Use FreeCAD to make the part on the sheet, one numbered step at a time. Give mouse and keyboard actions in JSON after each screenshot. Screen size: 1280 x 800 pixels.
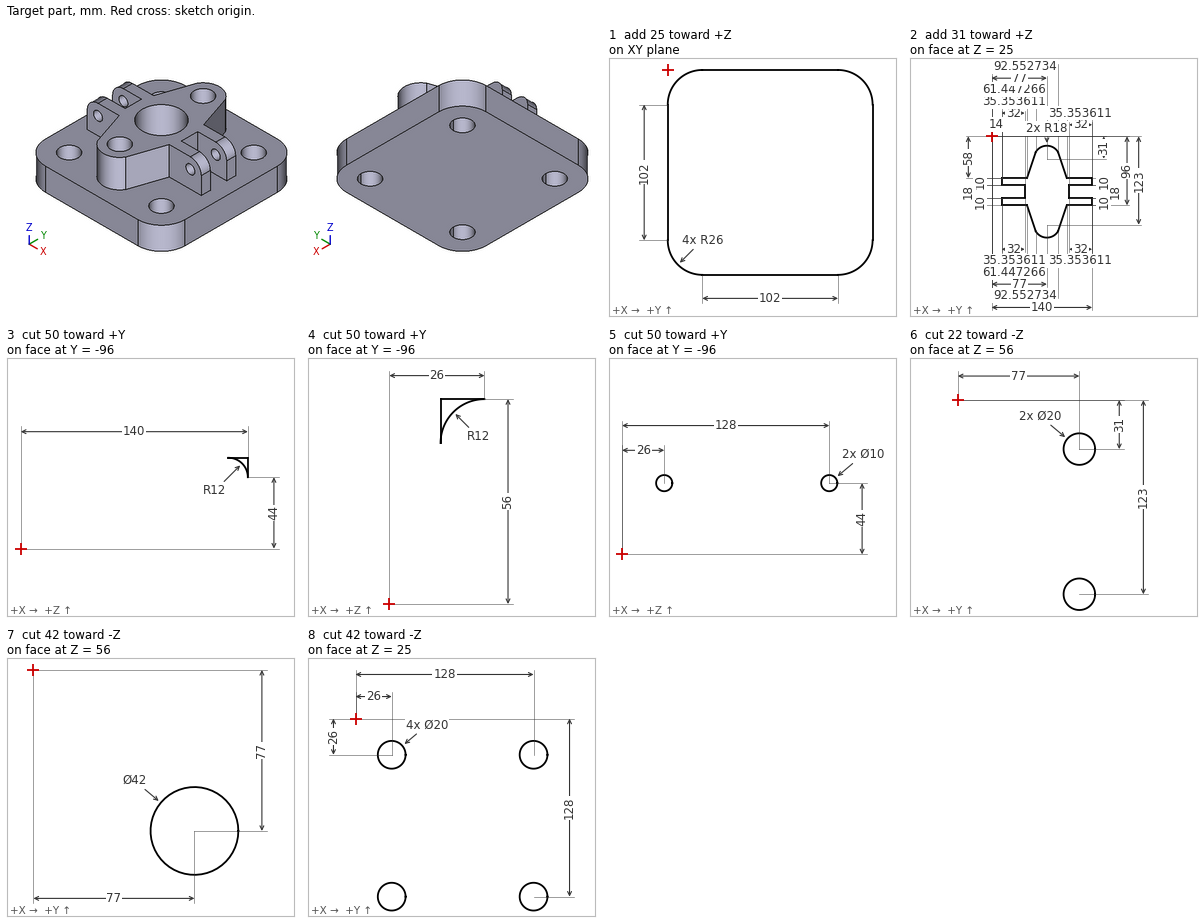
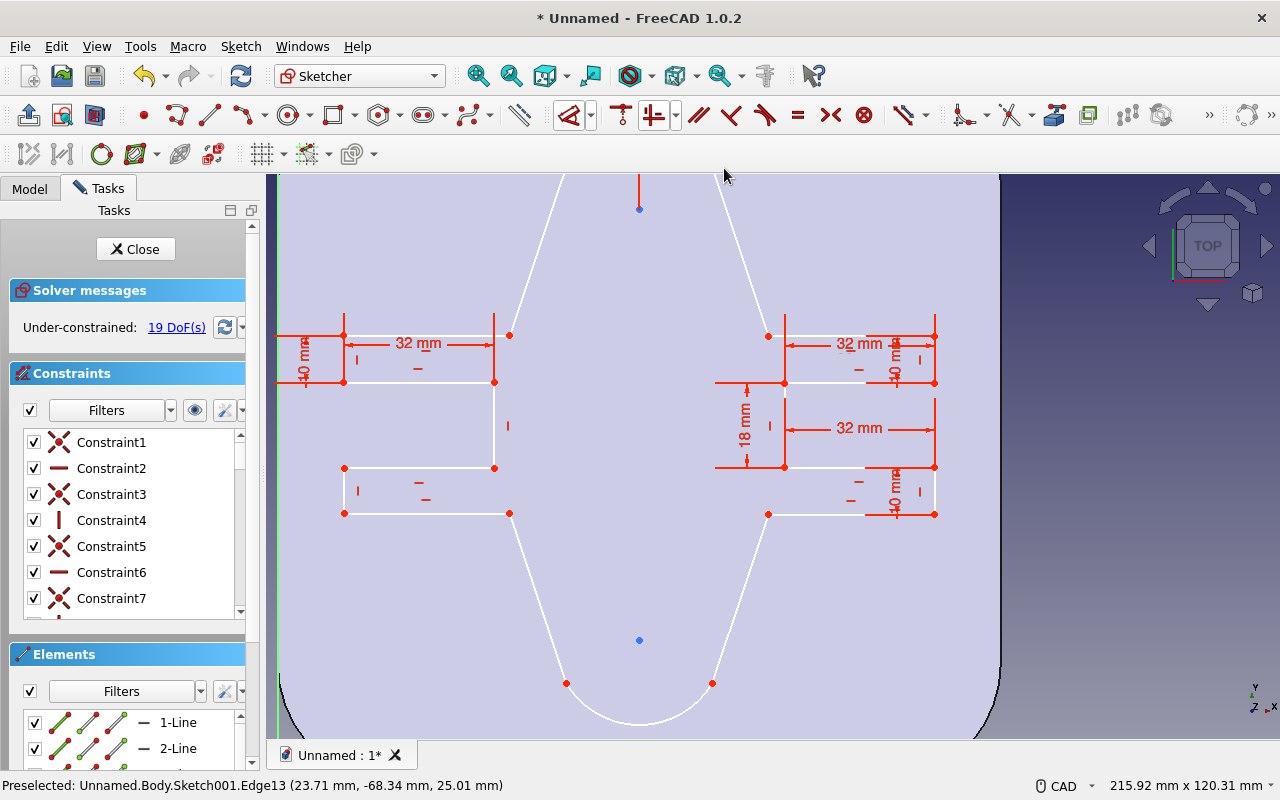
{"action": "left_click", "coordinate": [494, 408]}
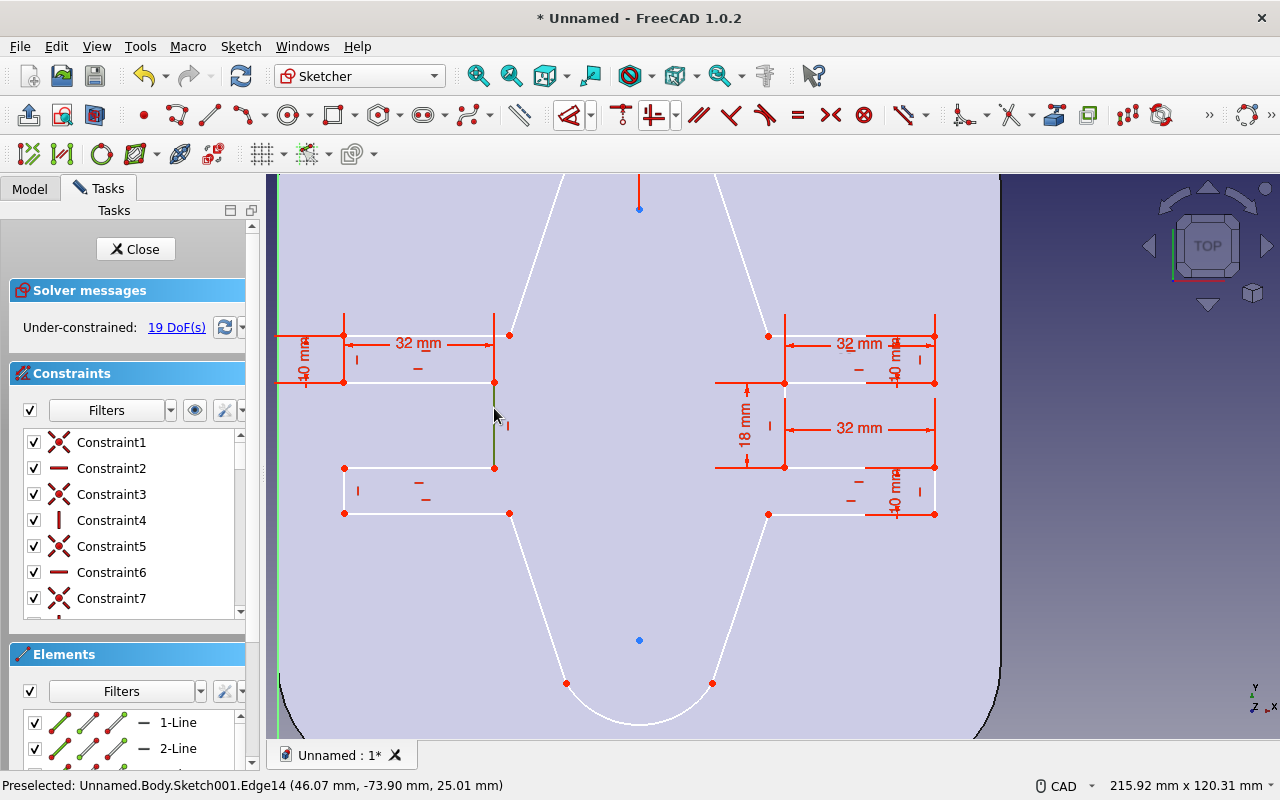
{"action": "left_click", "coordinate": [590, 116]}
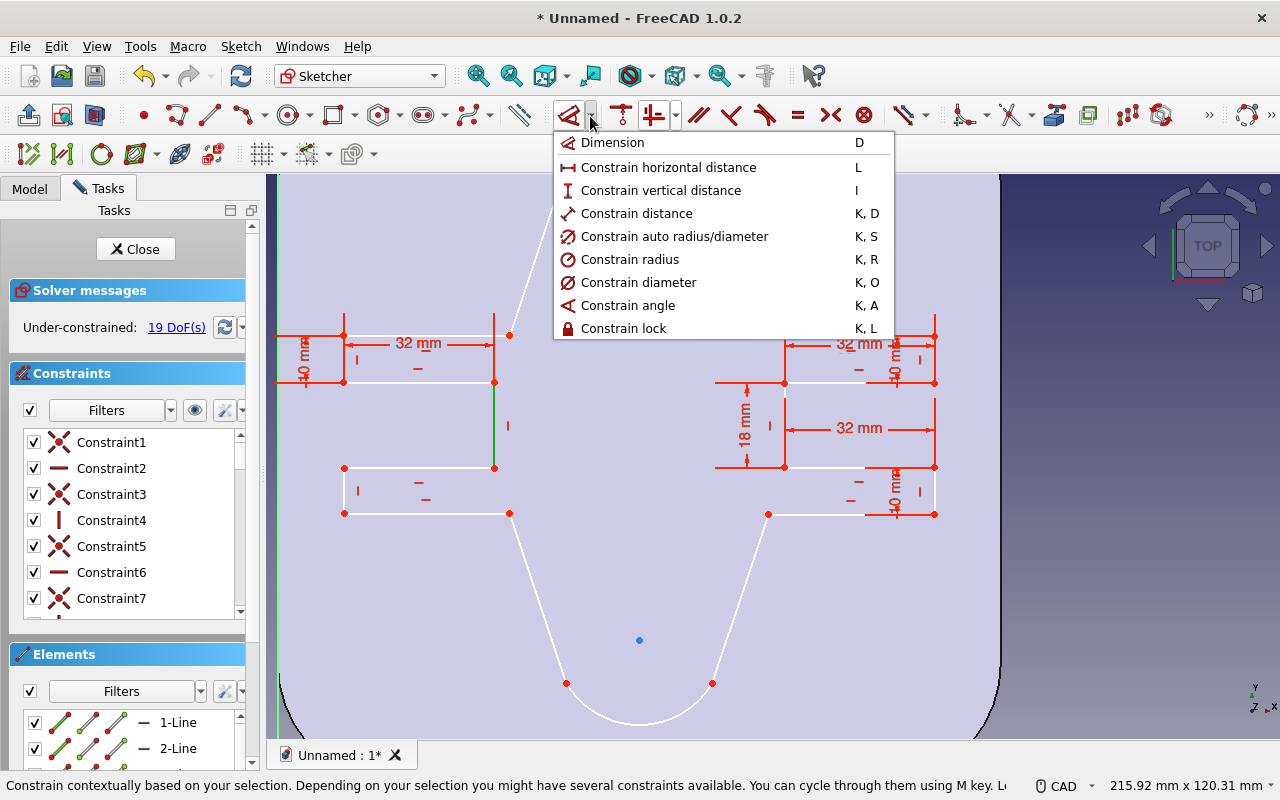
{"action": "left_click", "coordinate": [724, 190]}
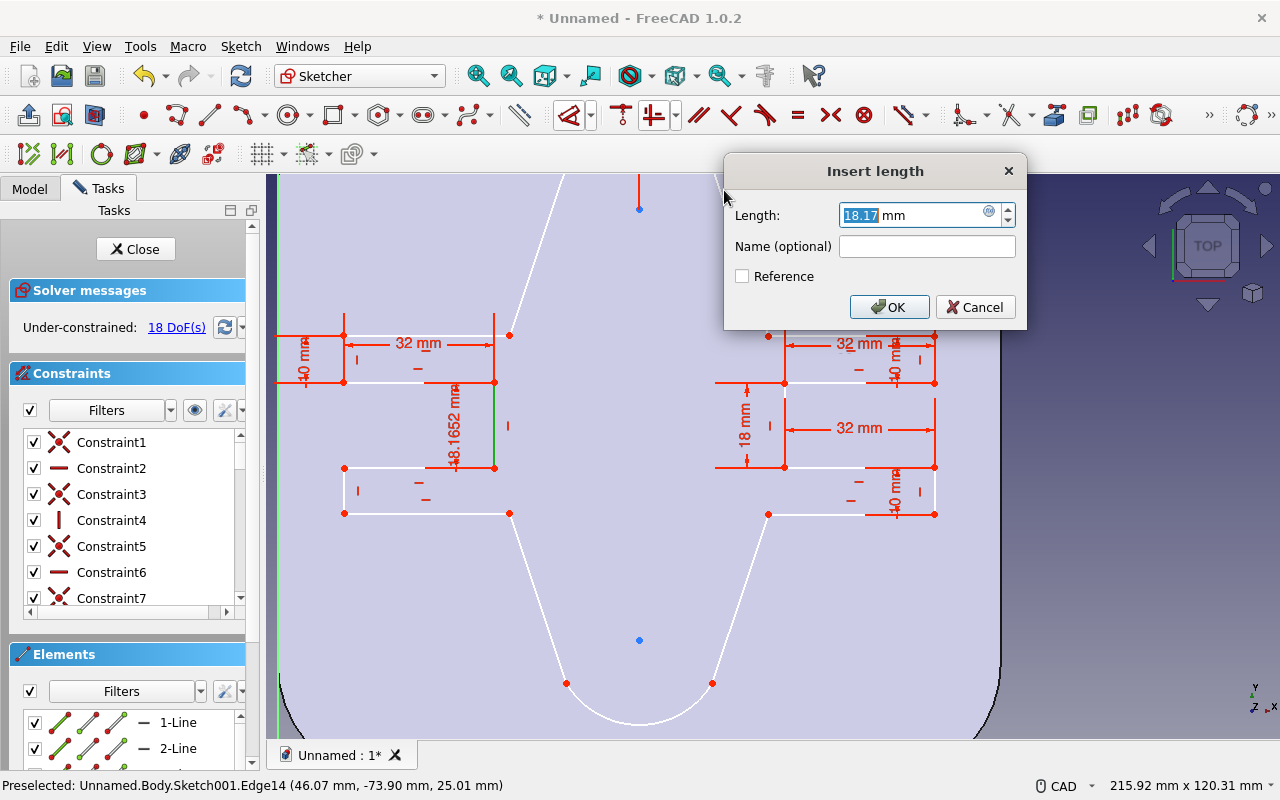
{"action": "type", "text": "18"}
{"action": "key", "text": "Return"}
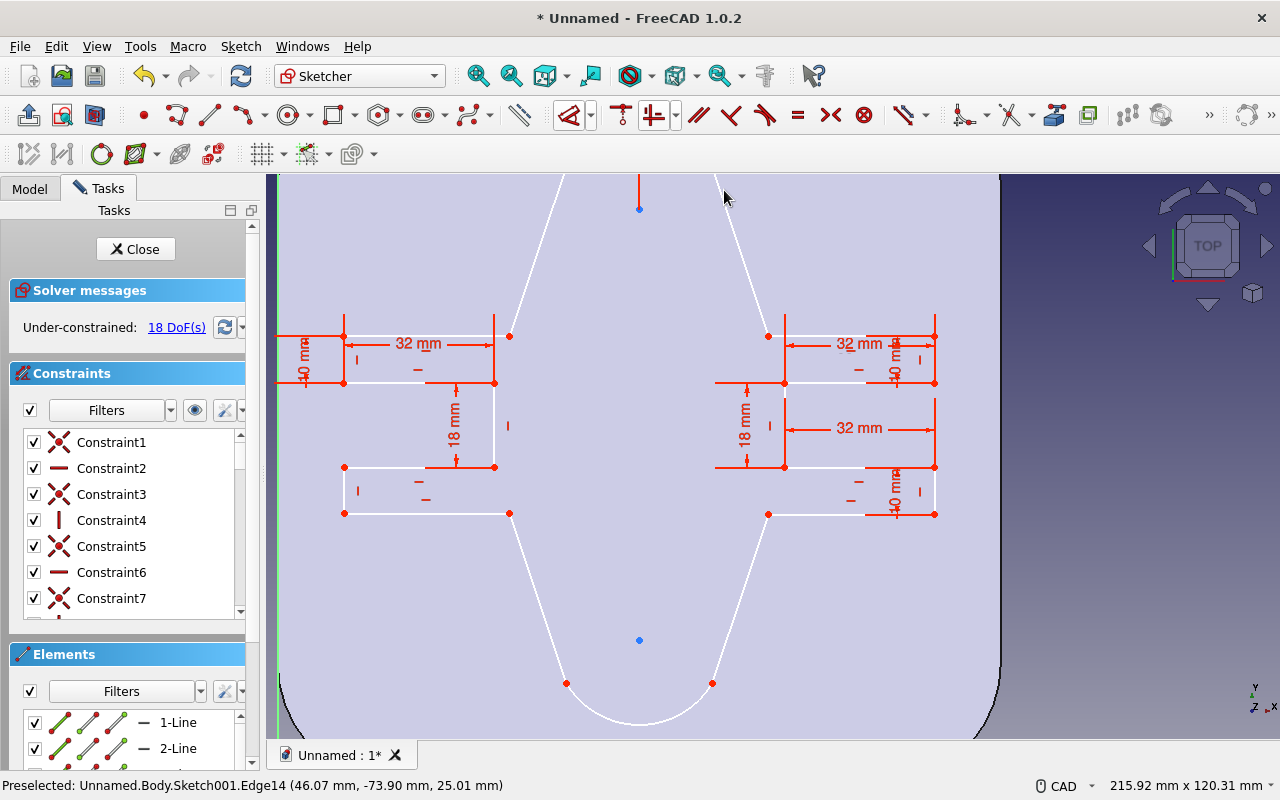
{"action": "left_click", "coordinate": [449, 468]}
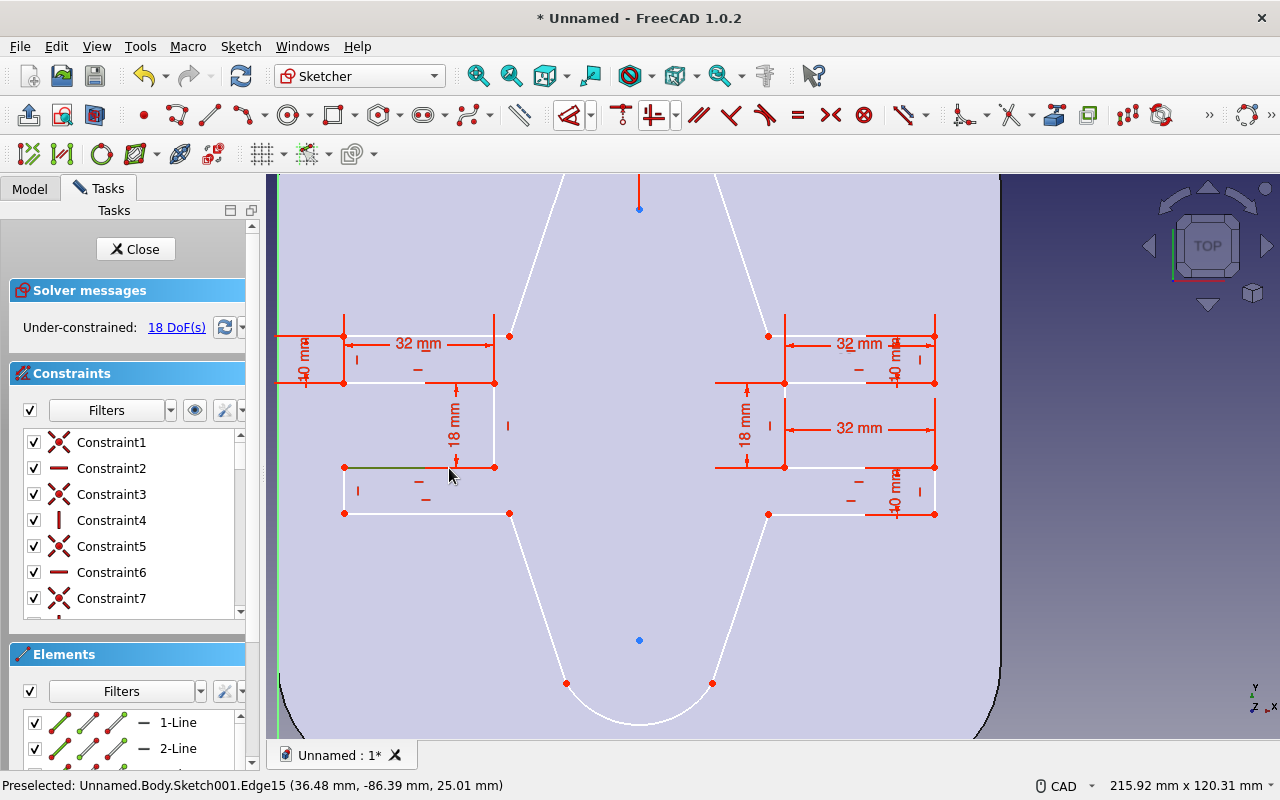
{"action": "key", "text": "l"}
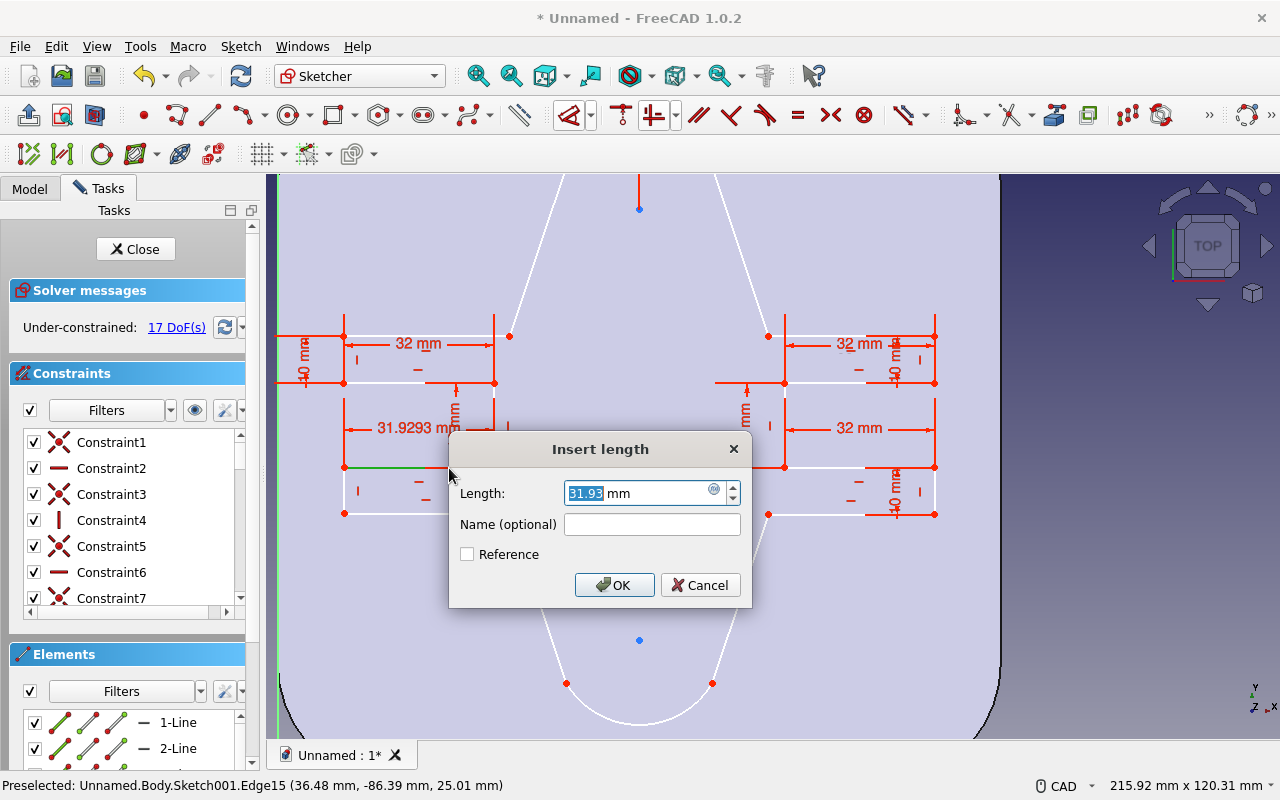
{"action": "type", "text": "32"}
{"action": "key", "text": "Return"}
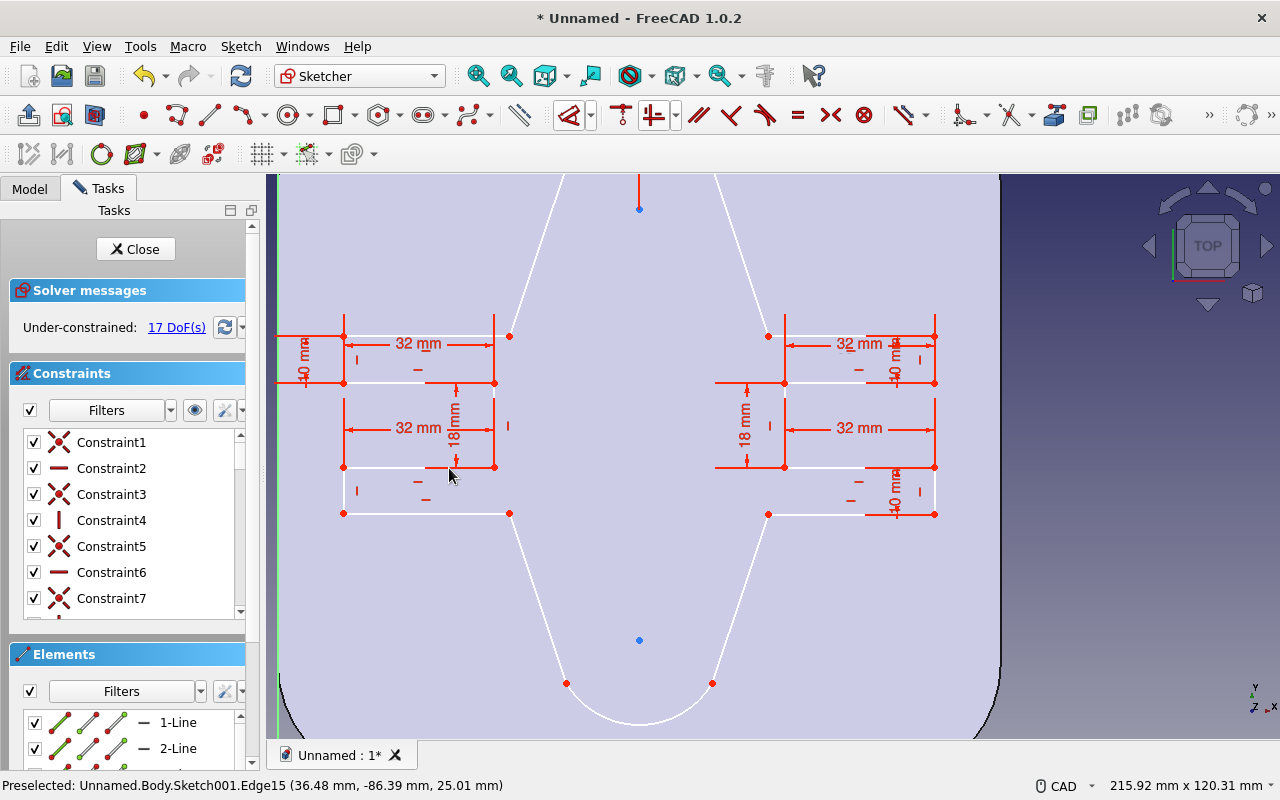
{"action": "left_click", "coordinate": [344, 481]}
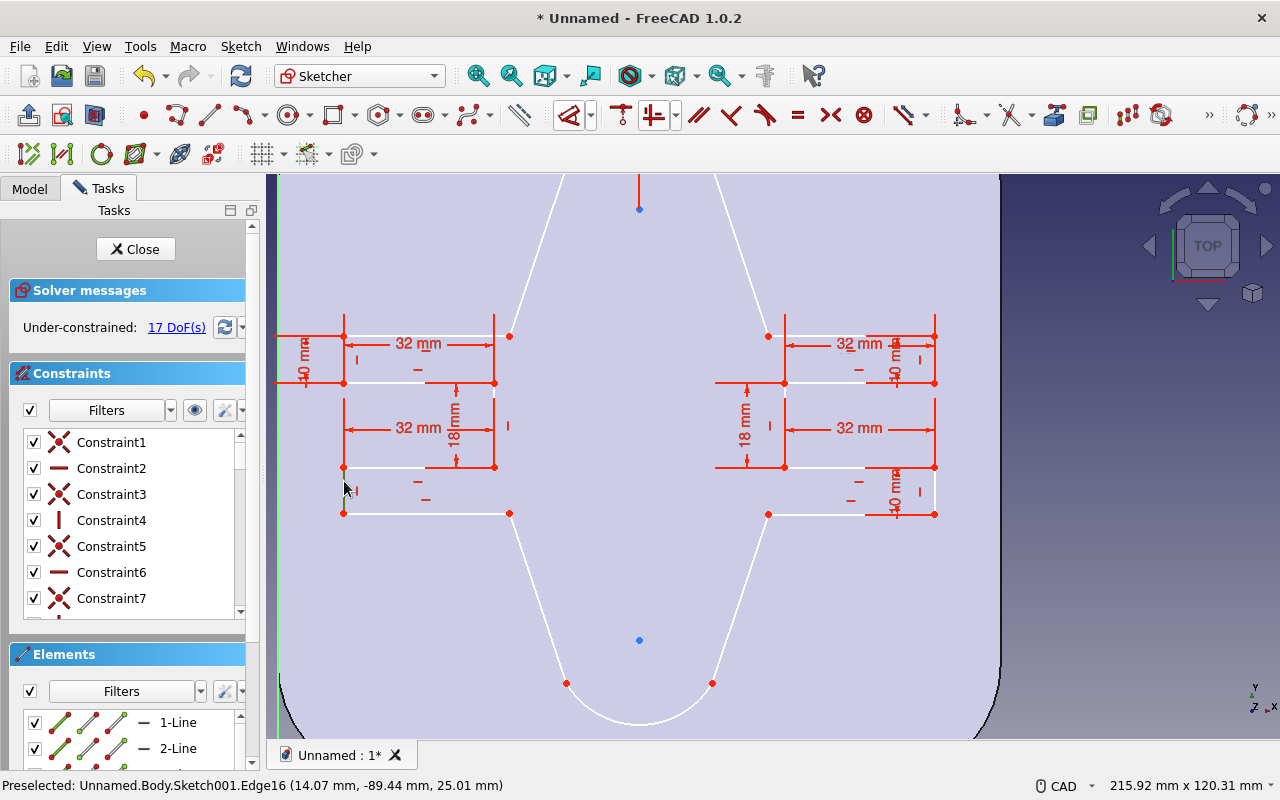
{"action": "left_click", "coordinate": [590, 116]}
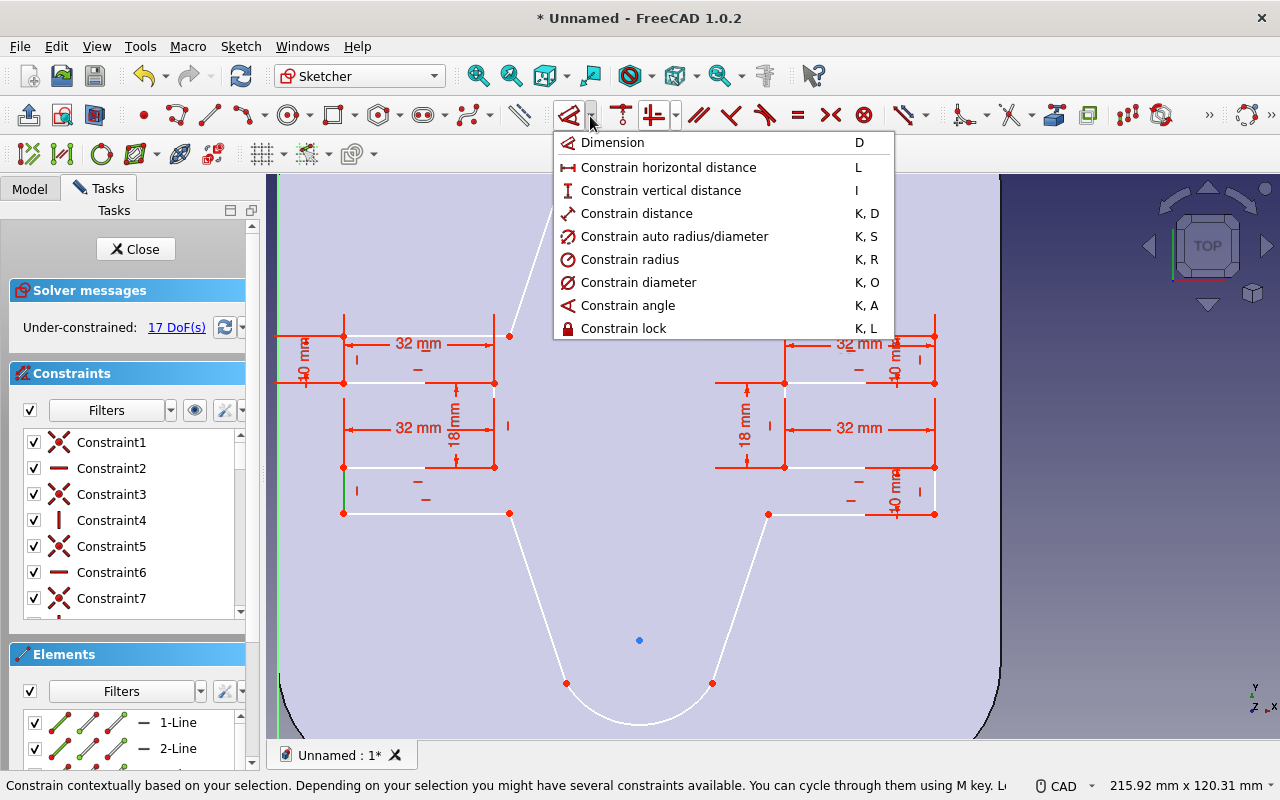
{"action": "left_click", "coordinate": [724, 190]}